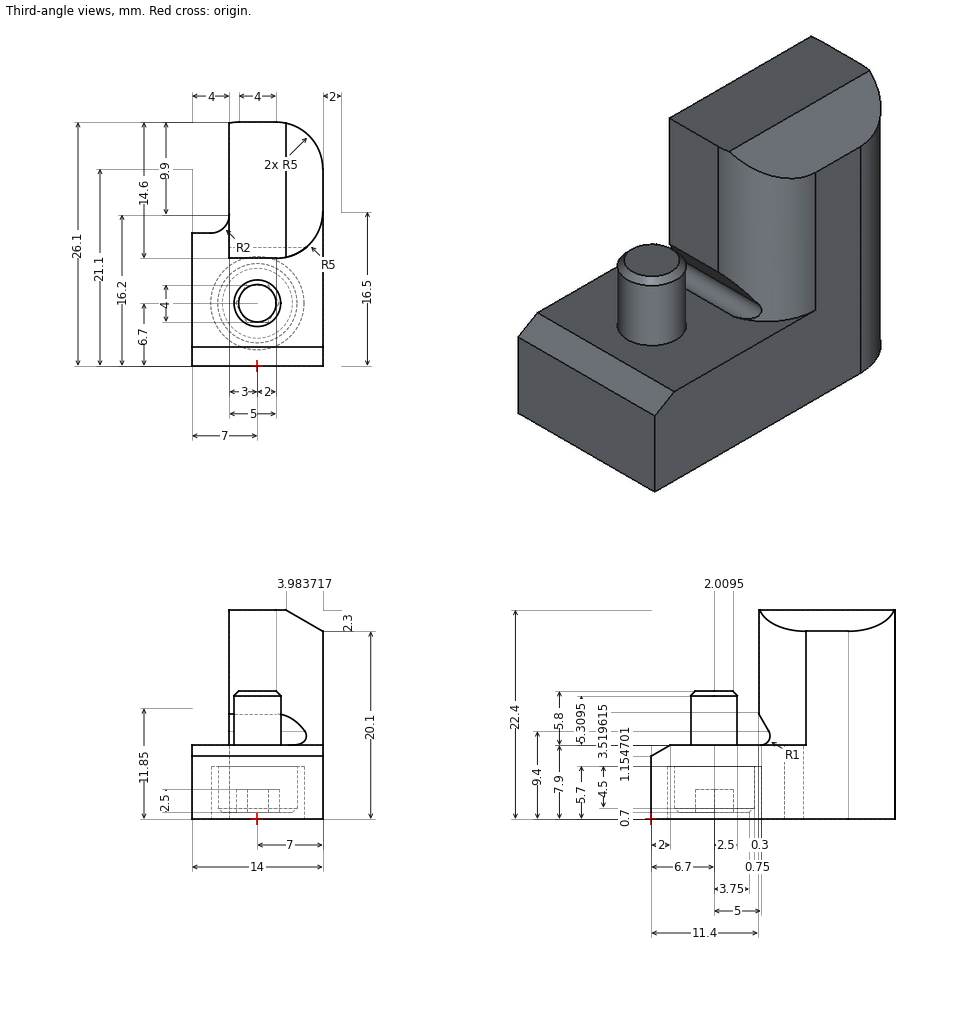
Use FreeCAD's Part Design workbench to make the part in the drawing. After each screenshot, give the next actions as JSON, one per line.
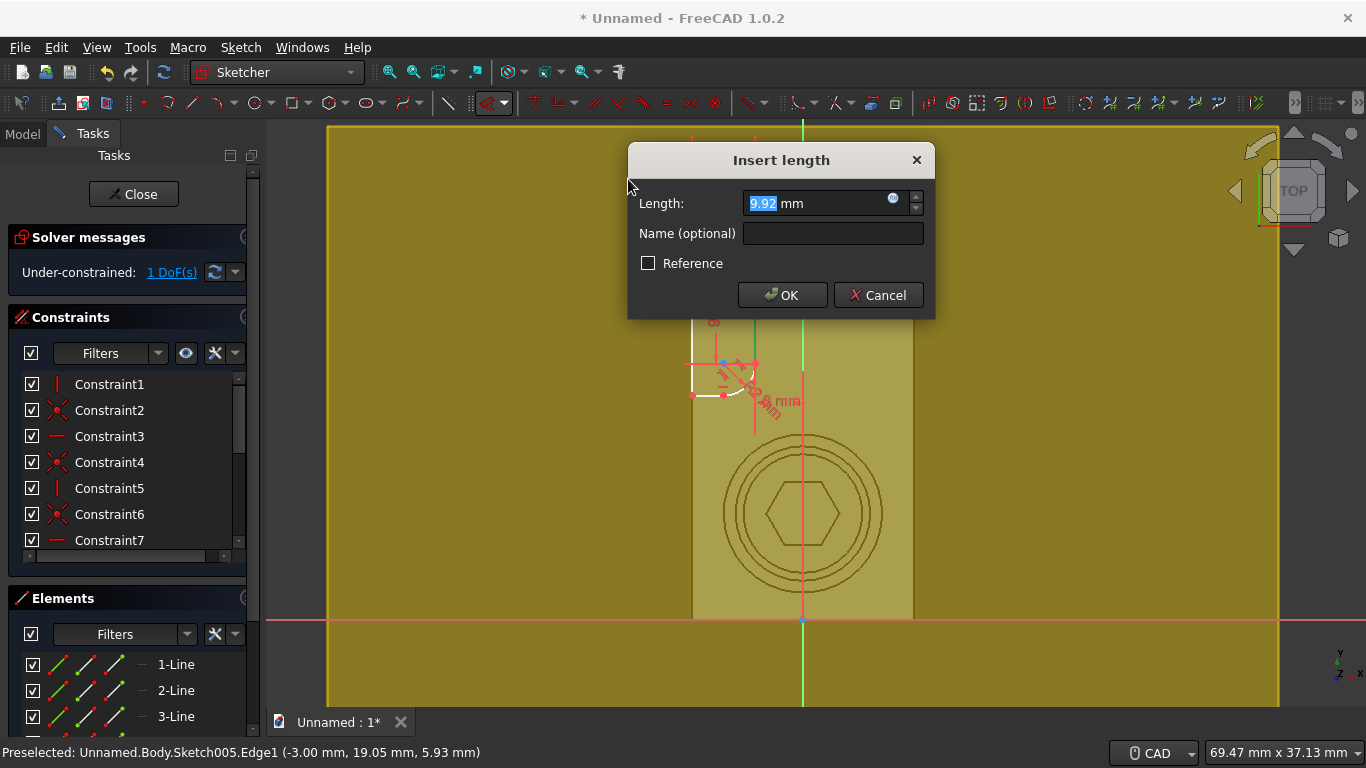
{"action": "type", "text": "9.9"}
{"action": "key", "text": "Return"}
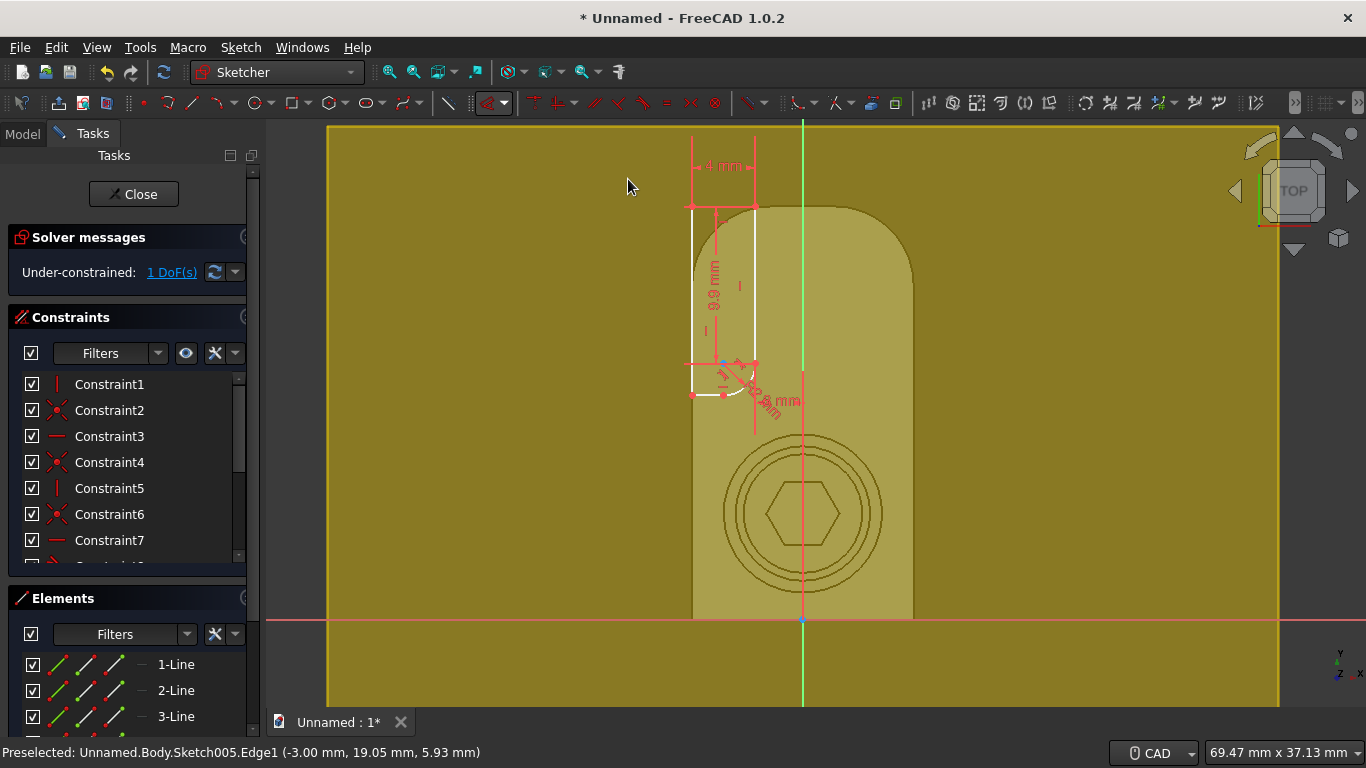
{"action": "left_click", "coordinate": [755, 364]}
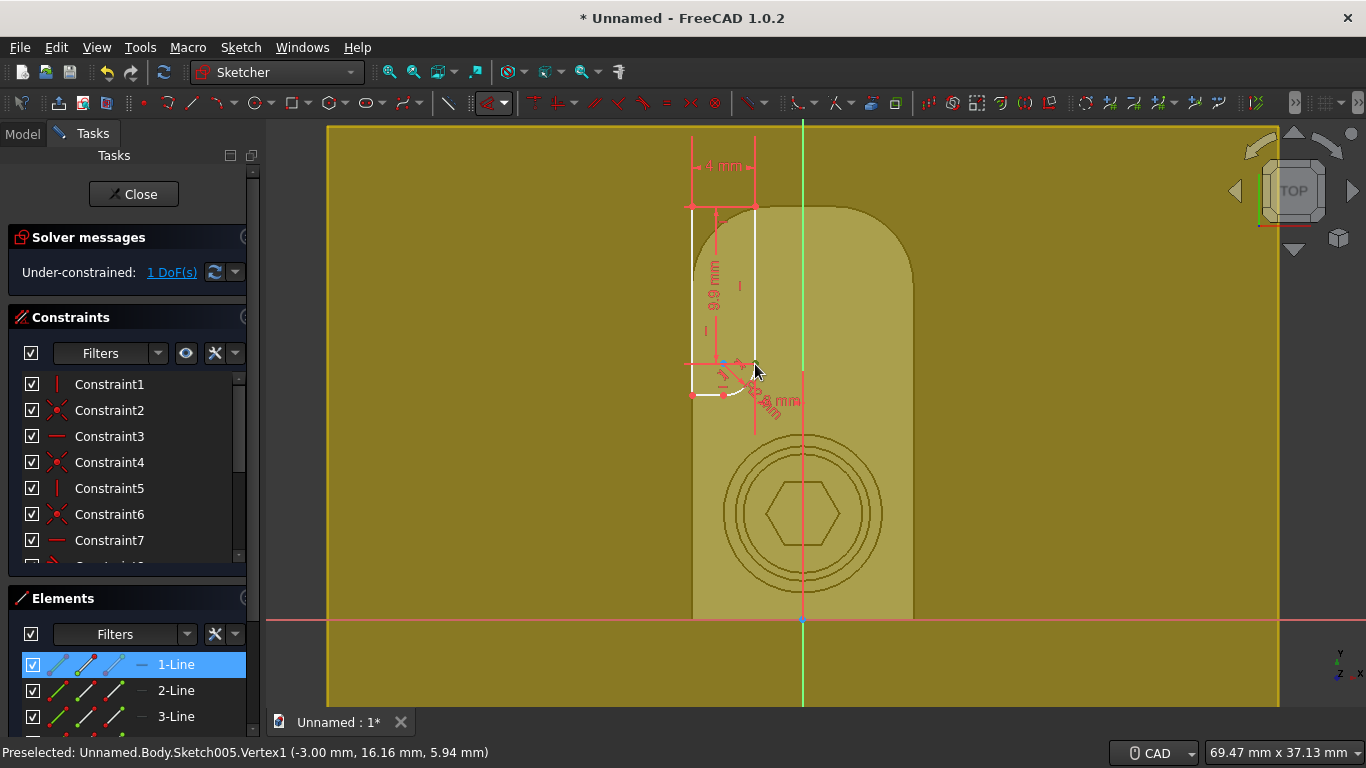
{"action": "left_click", "coordinate": [506, 104]}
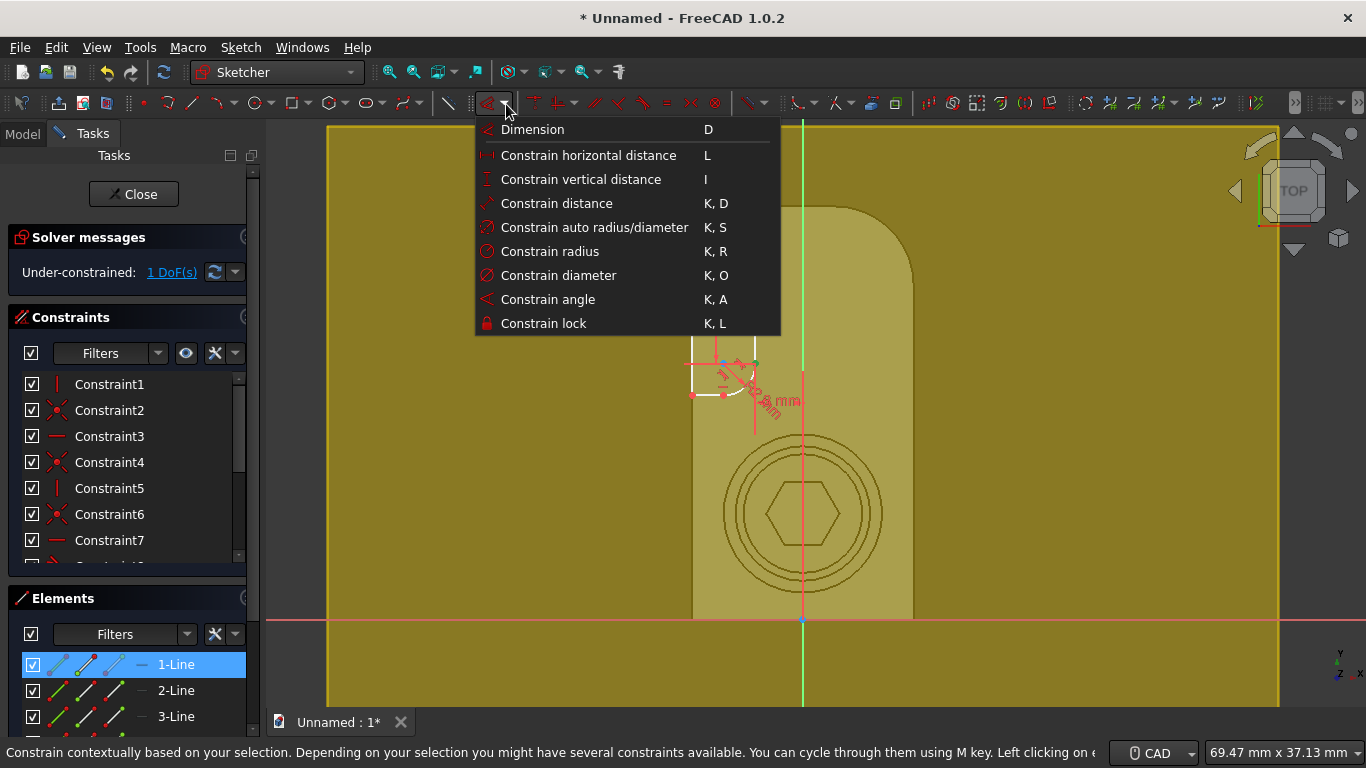
{"action": "left_click", "coordinate": [628, 179]}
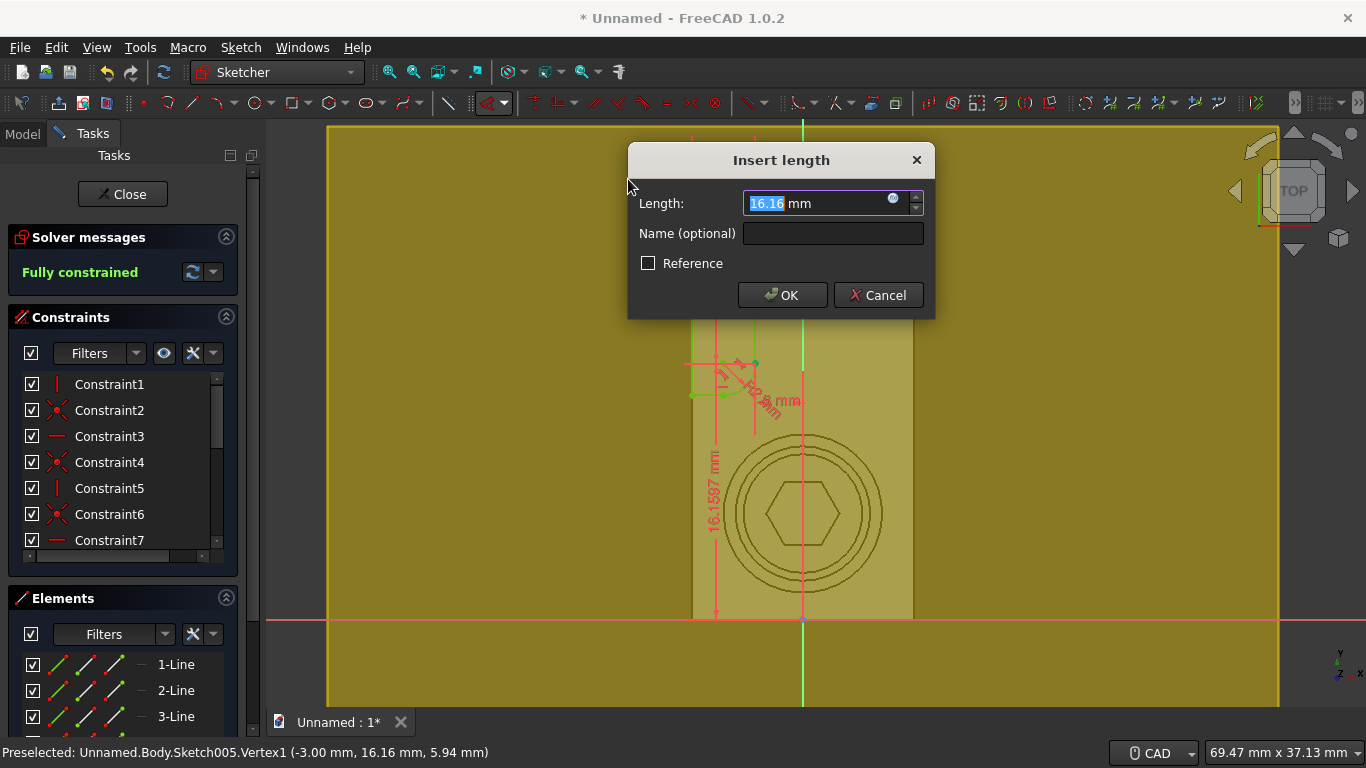
{"action": "type", "text": "16.2"}
{"action": "key", "text": "Return"}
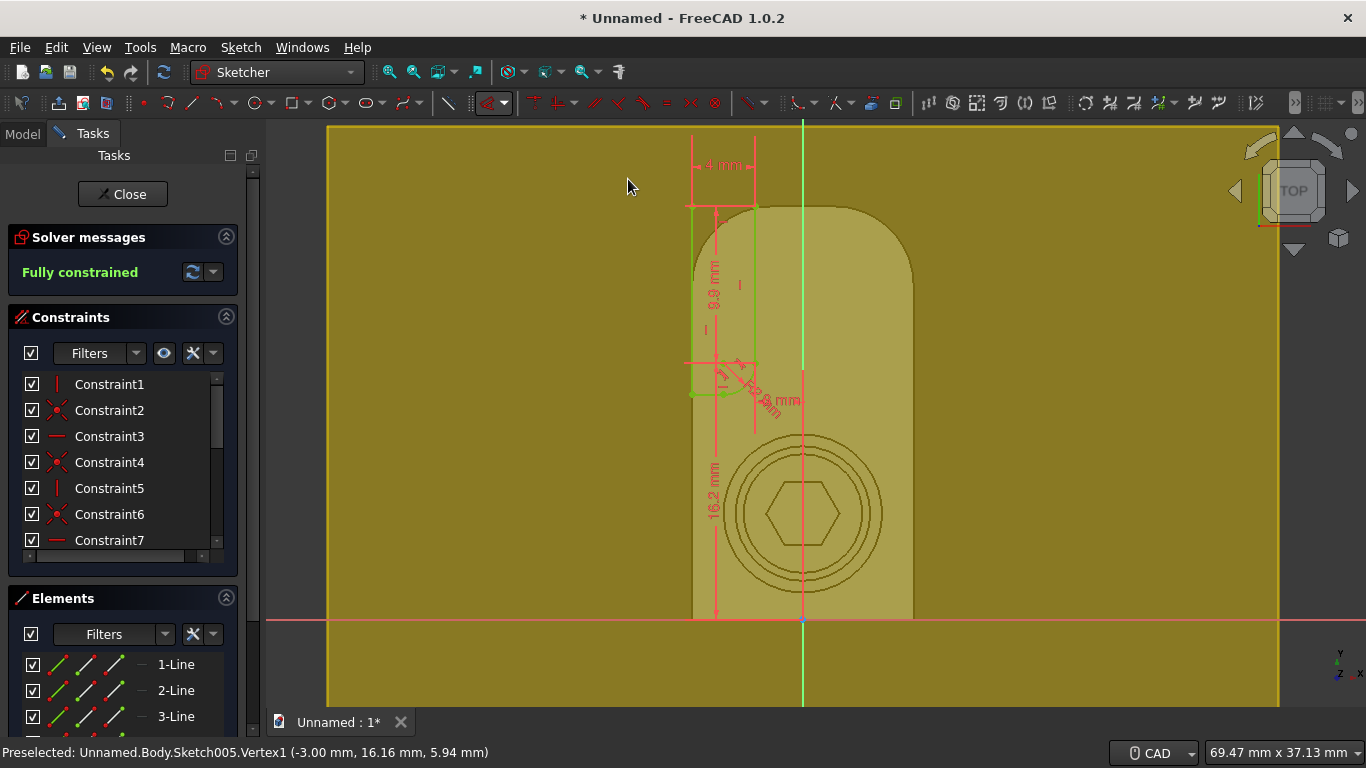
{"action": "left_click", "coordinate": [123, 194]}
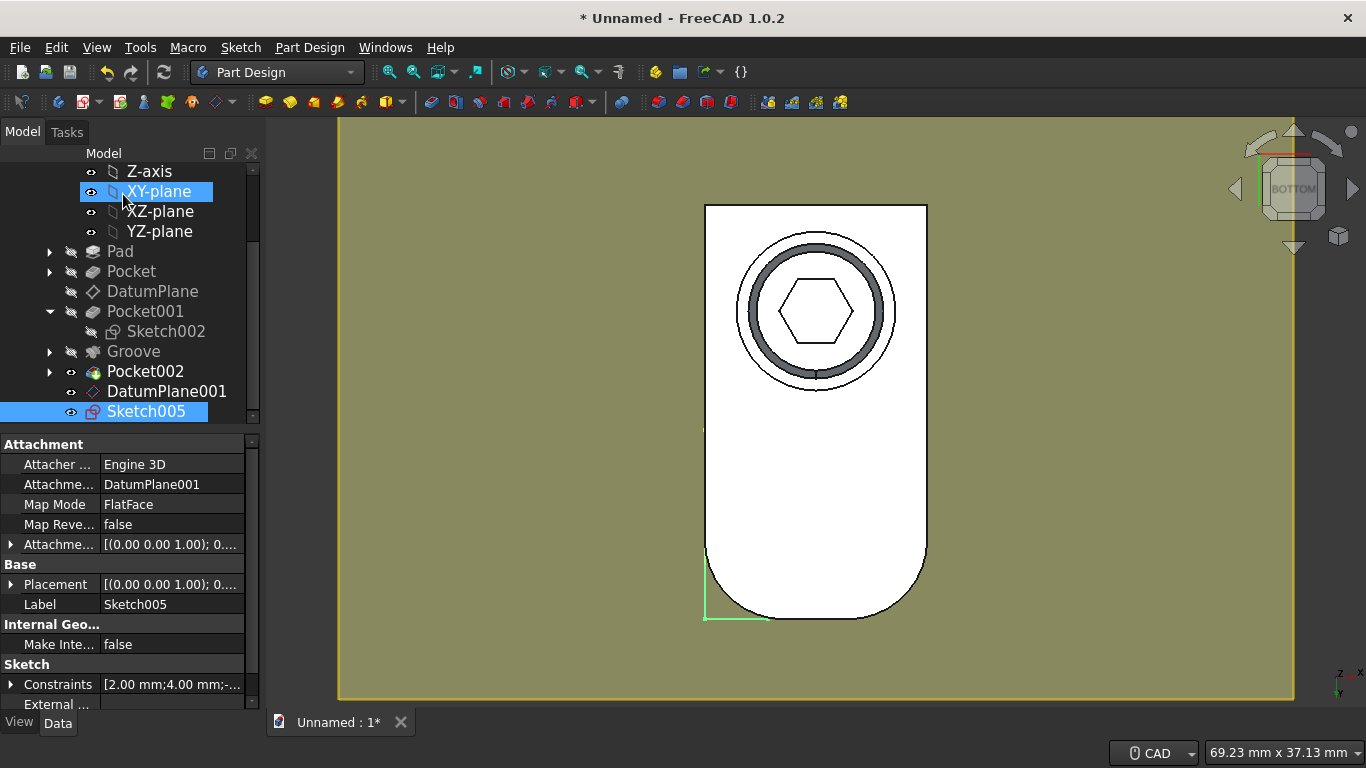
{"action": "left_click", "coordinate": [432, 102]}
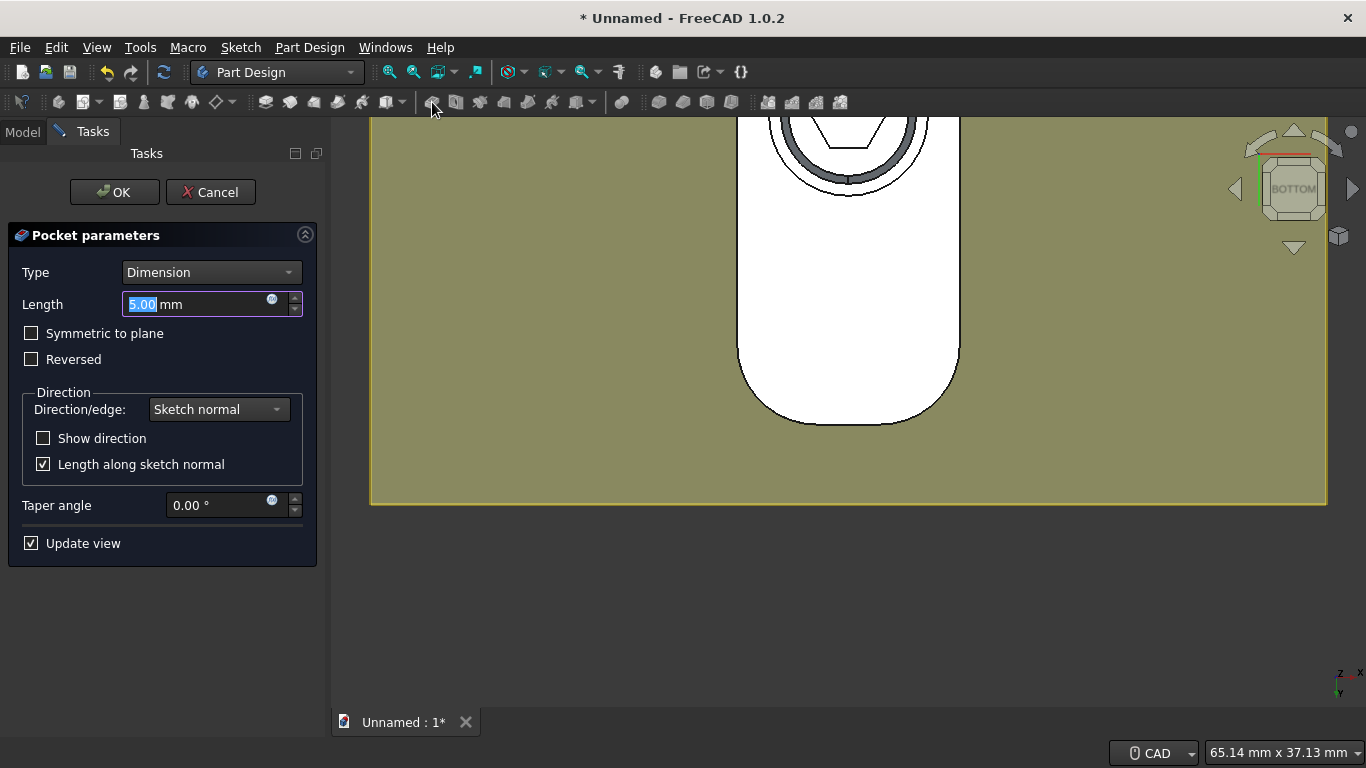
{"action": "type", "text": "11.85"}
{"action": "key", "text": "Tab"}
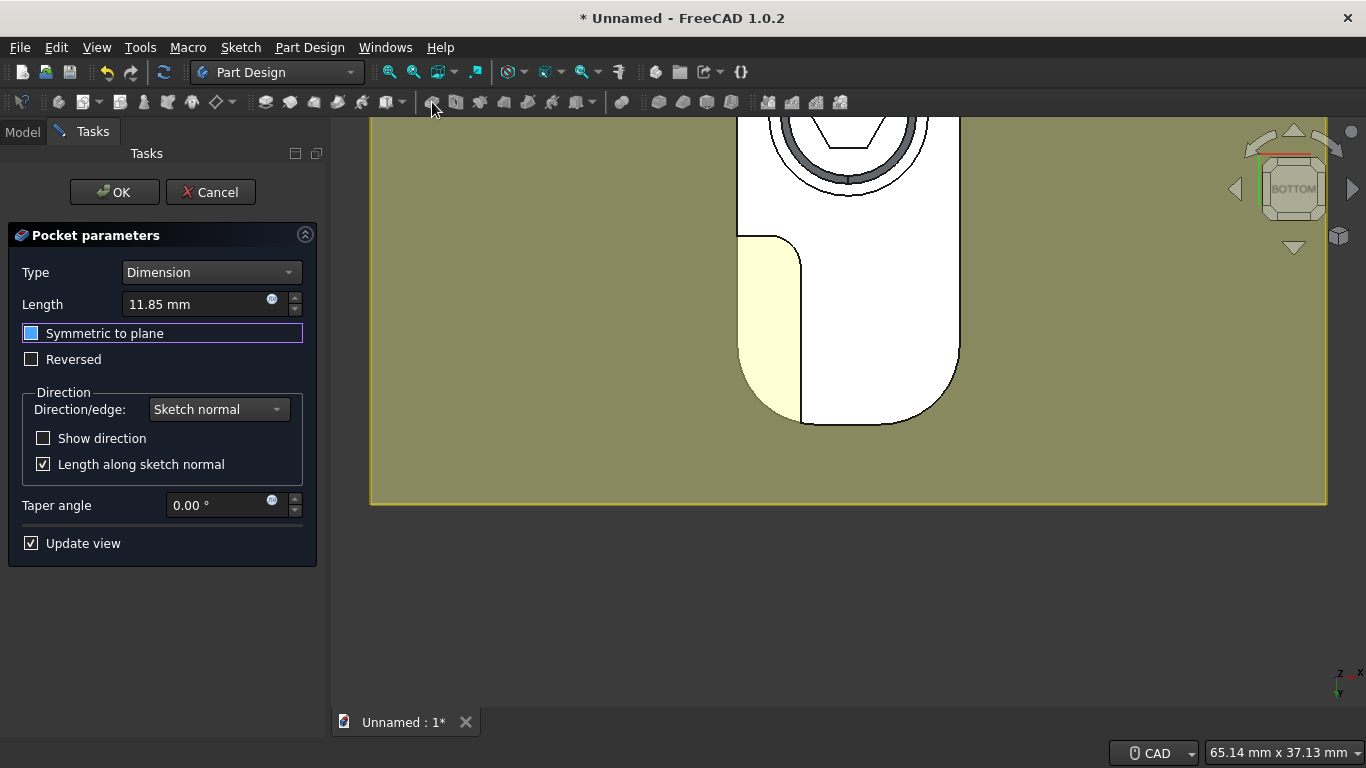
{"action": "left_click", "coordinate": [30, 333]}